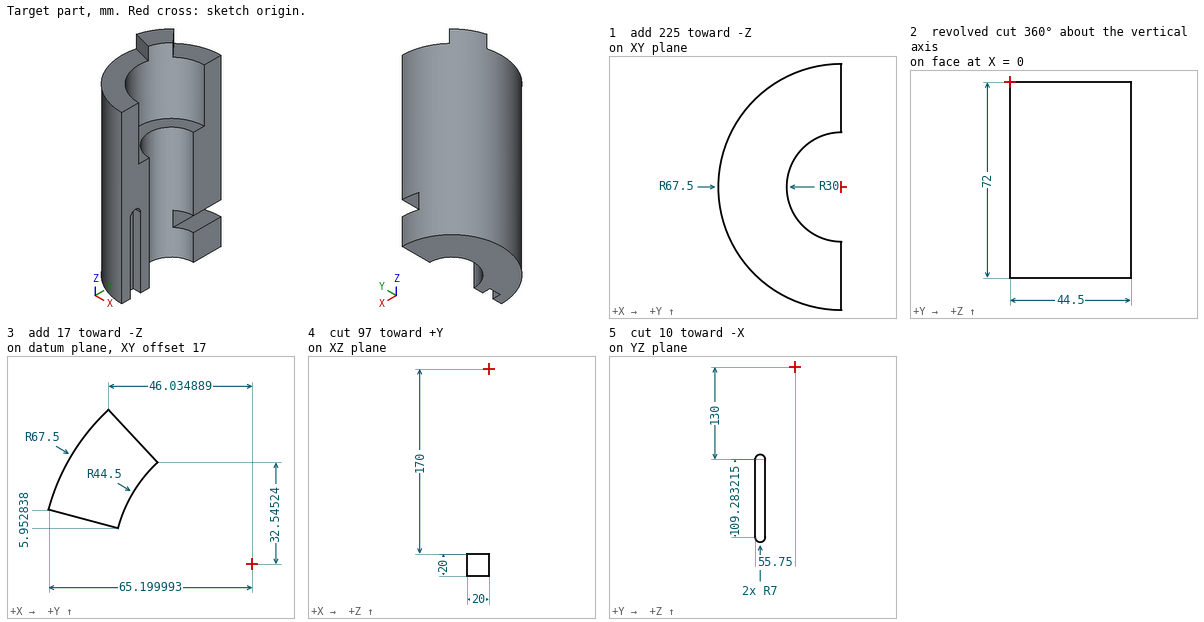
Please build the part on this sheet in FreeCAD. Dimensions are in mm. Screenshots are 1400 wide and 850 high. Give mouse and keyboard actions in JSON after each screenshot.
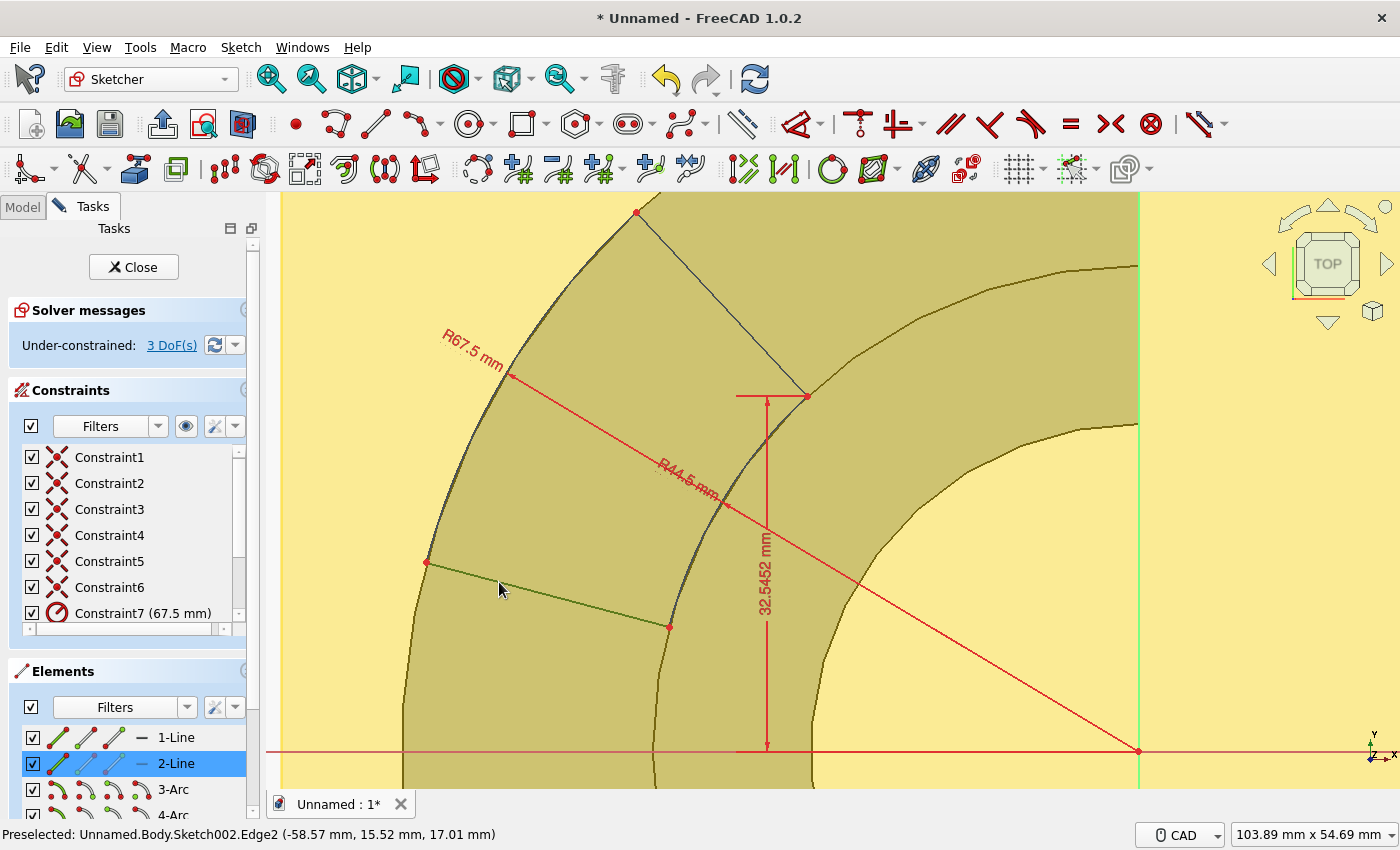
{"action": "key", "text": "i"}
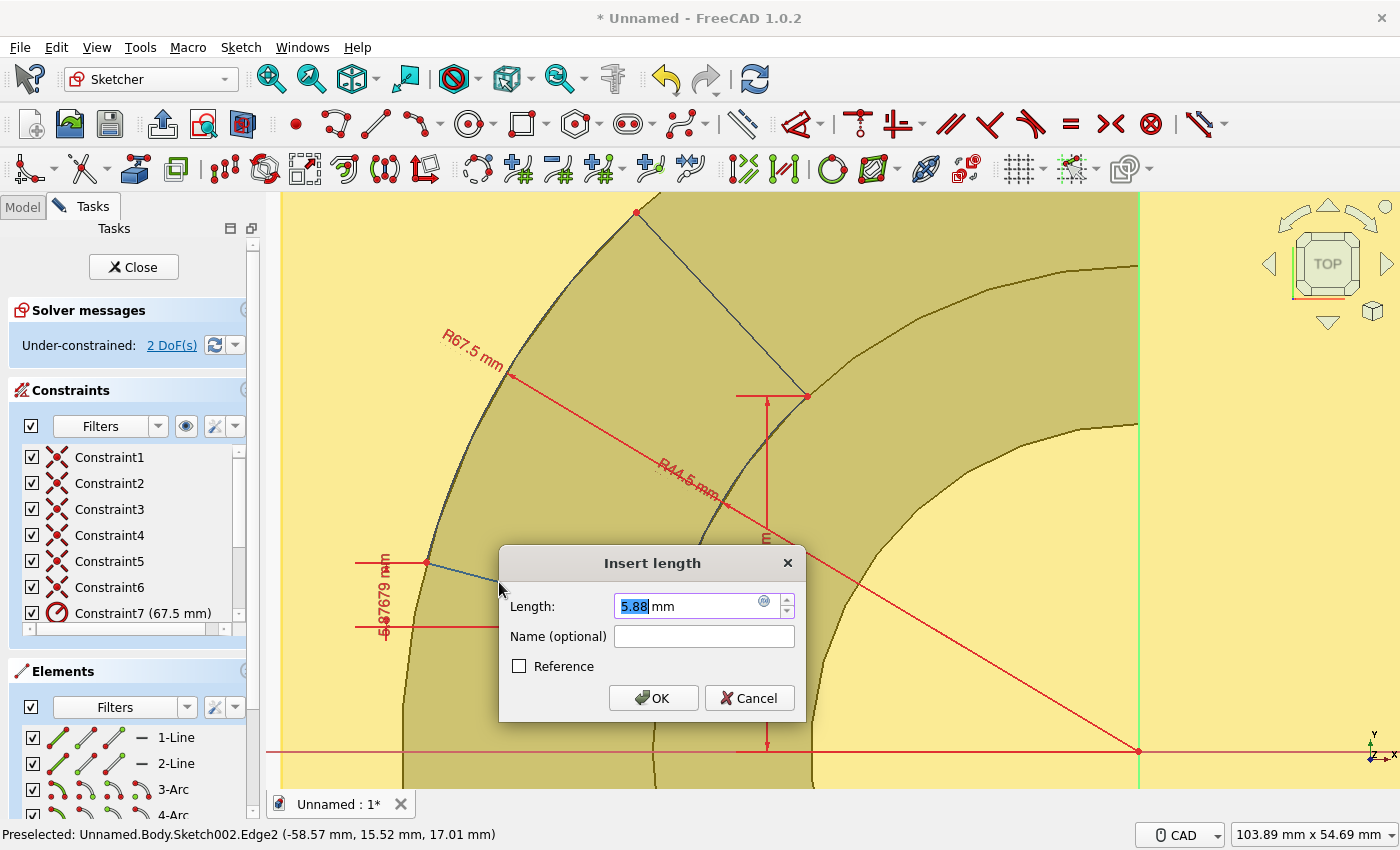
{"action": "type", "text": "5.952838"}
{"action": "key", "text": "Return"}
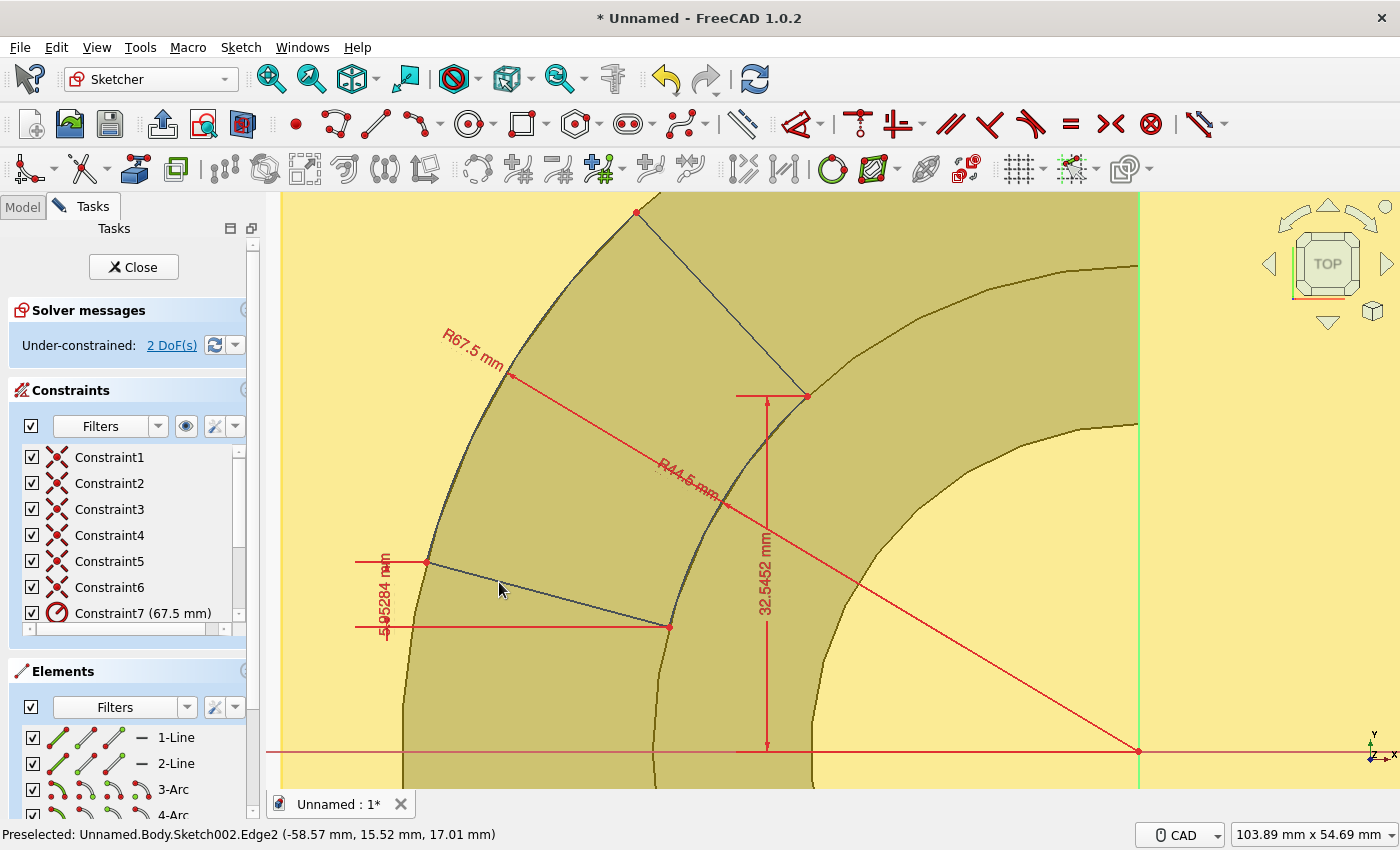
{"action": "scroll", "coordinate": [728, 508], "scroll_direction": "down", "scroll_amount": 2}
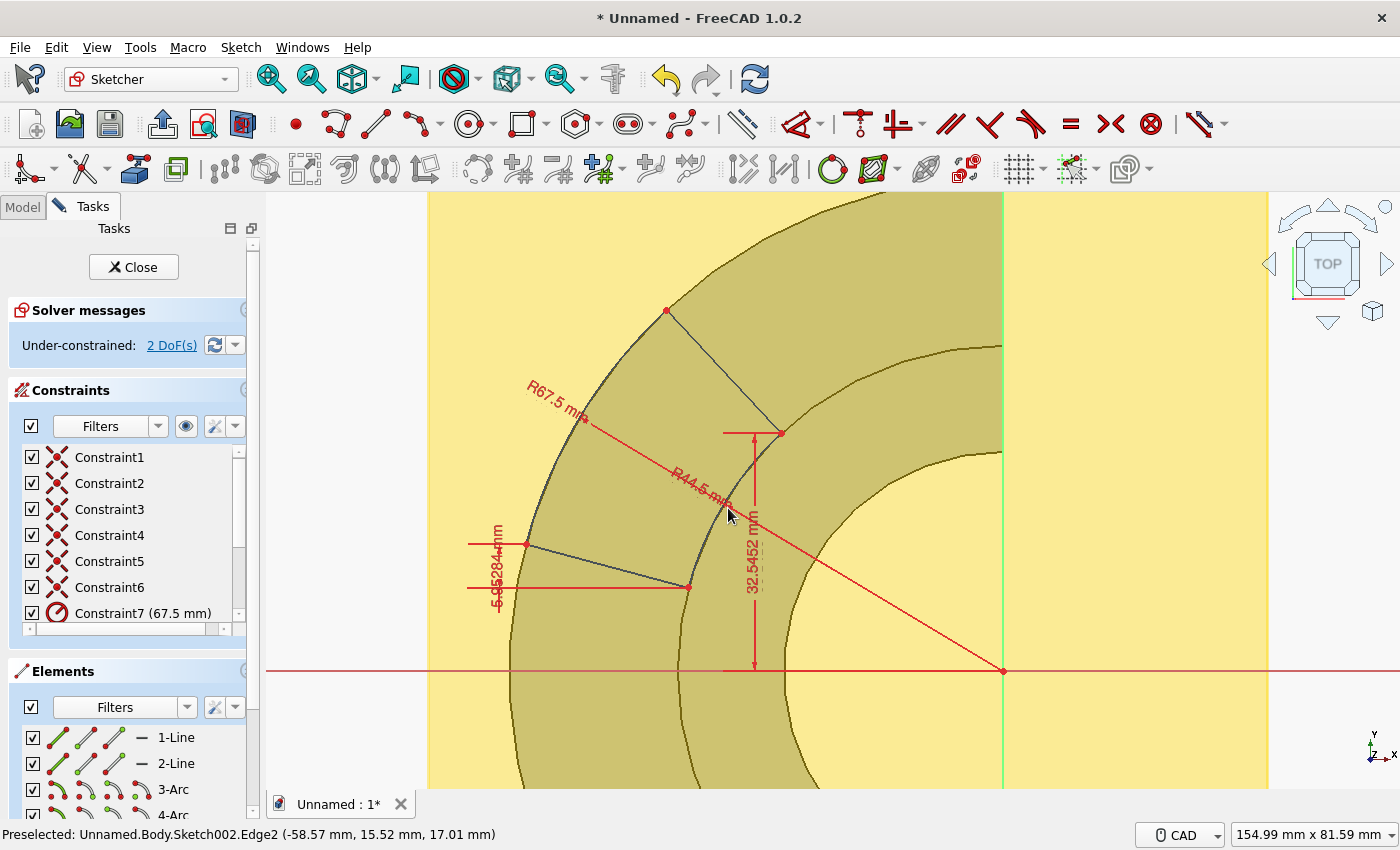
{"action": "left_click", "coordinate": [667, 310]}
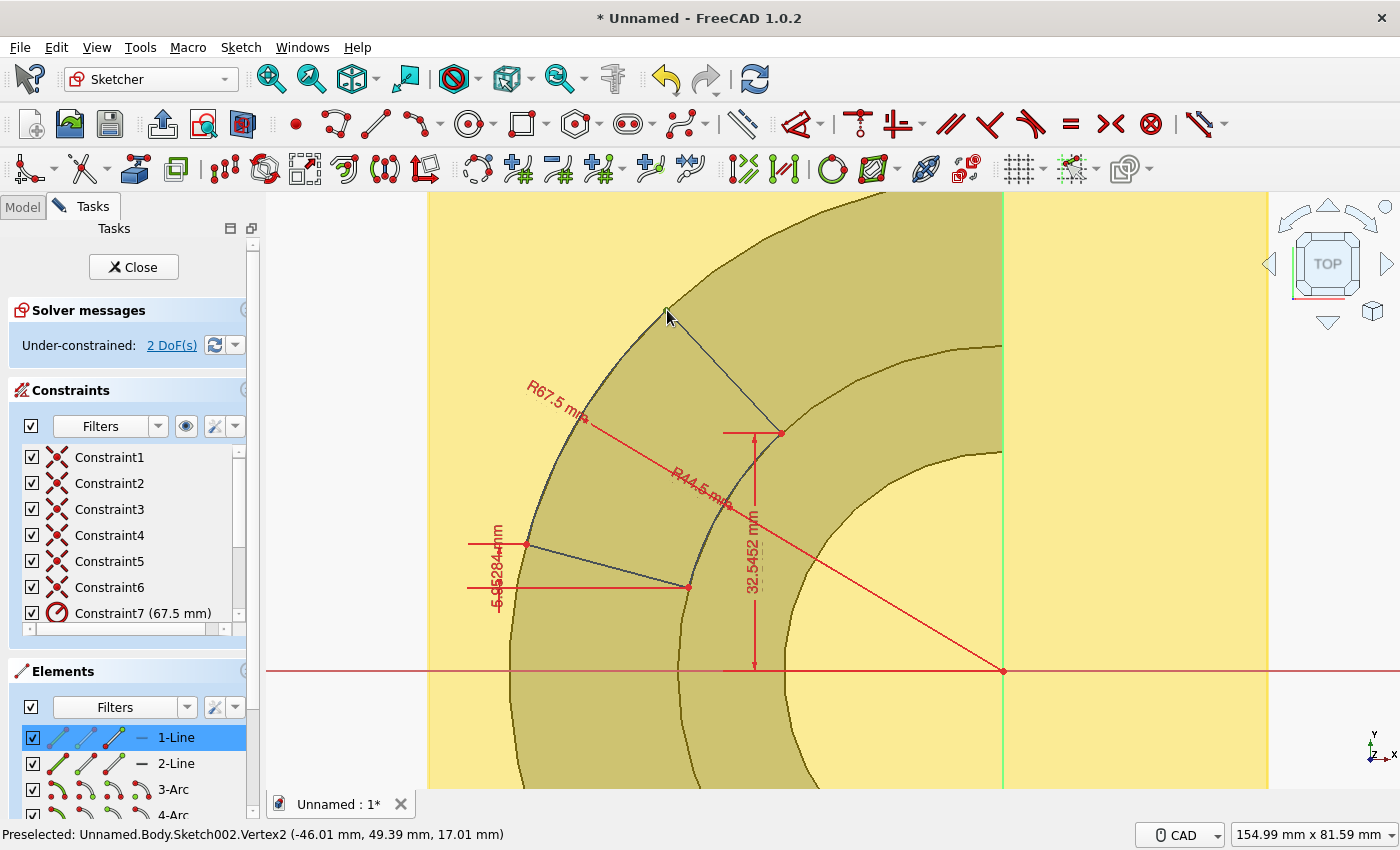
{"action": "left_click", "coordinate": [822, 124]}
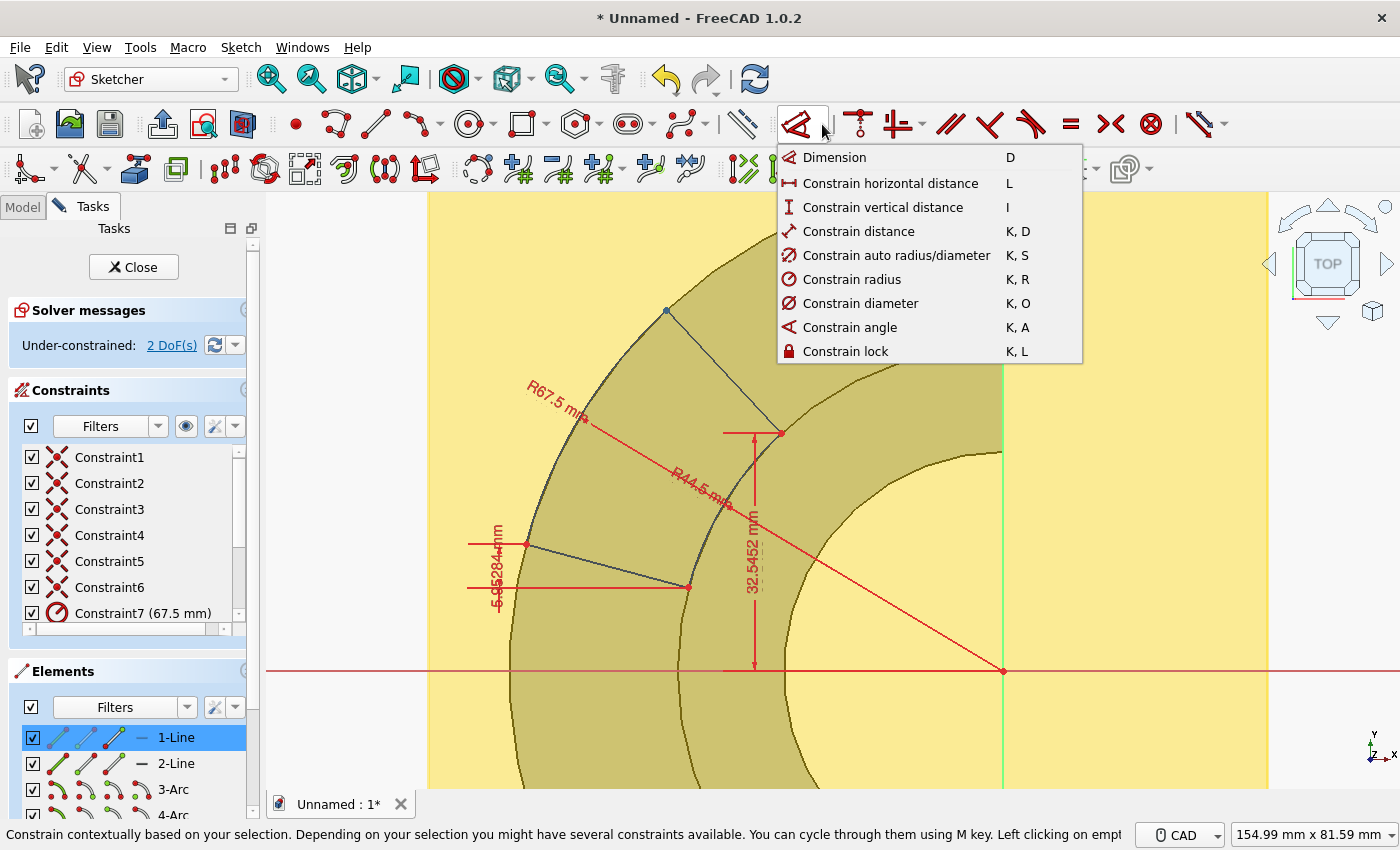
{"action": "left_click", "coordinate": [930, 183]}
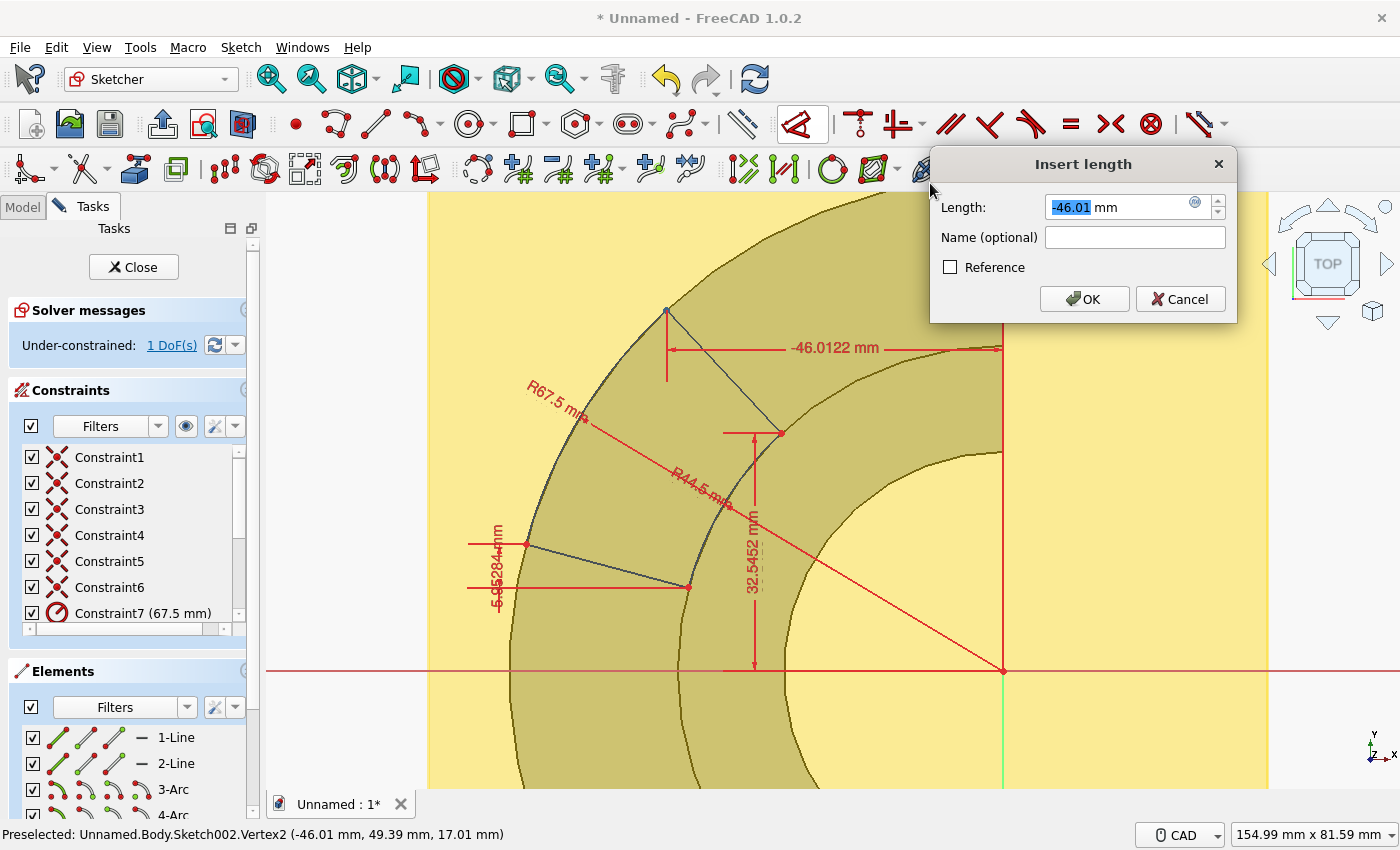
{"action": "type", "text": "-46.034889"}
{"action": "key", "text": "Return"}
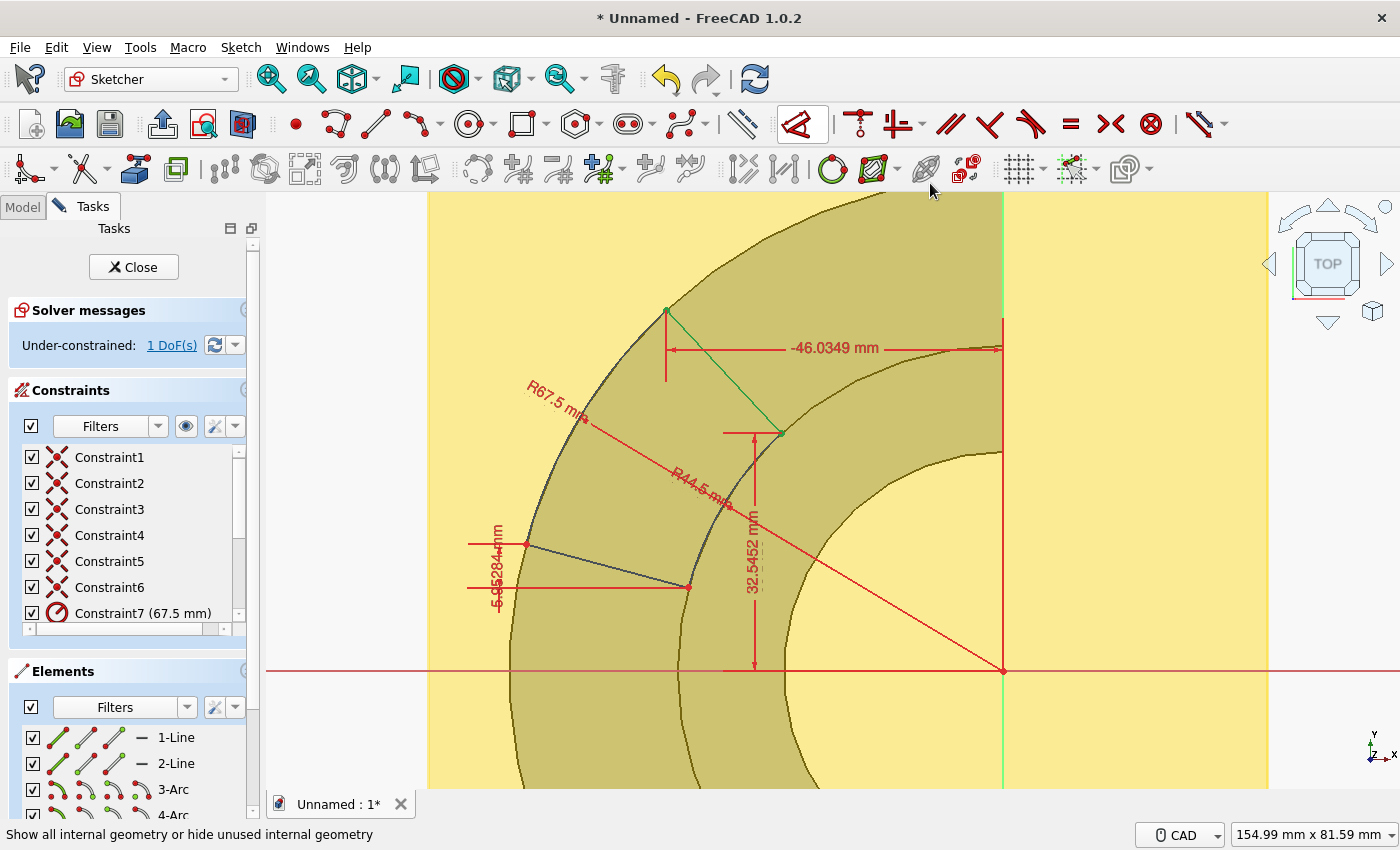
{"action": "left_click", "coordinate": [526, 544]}